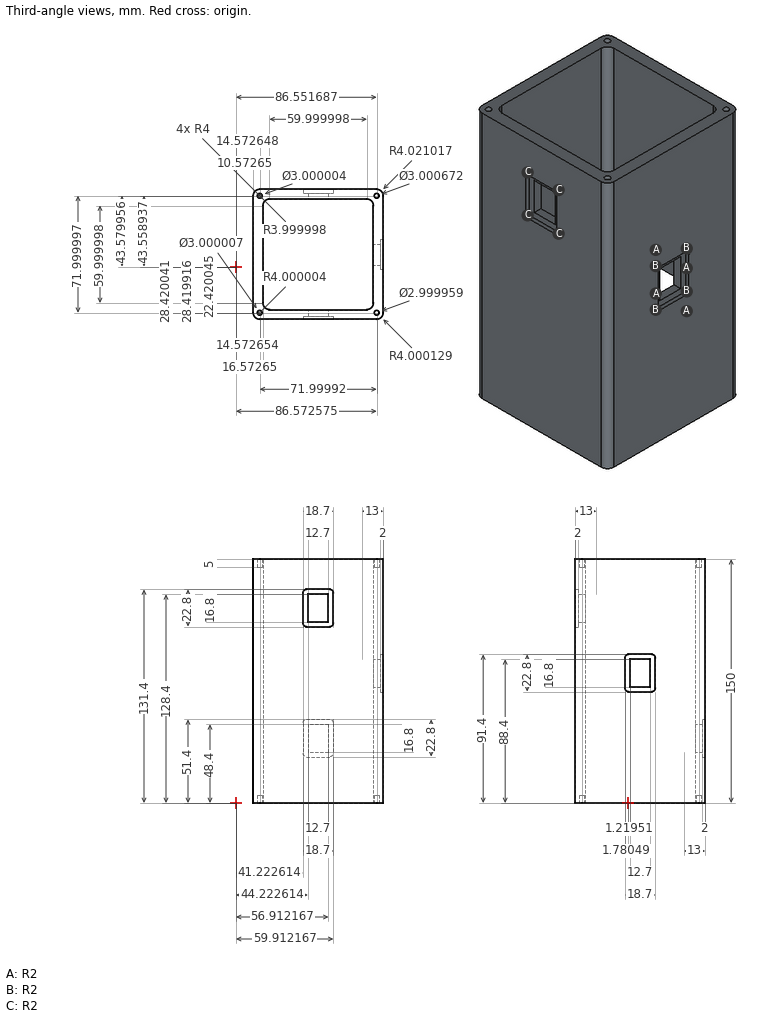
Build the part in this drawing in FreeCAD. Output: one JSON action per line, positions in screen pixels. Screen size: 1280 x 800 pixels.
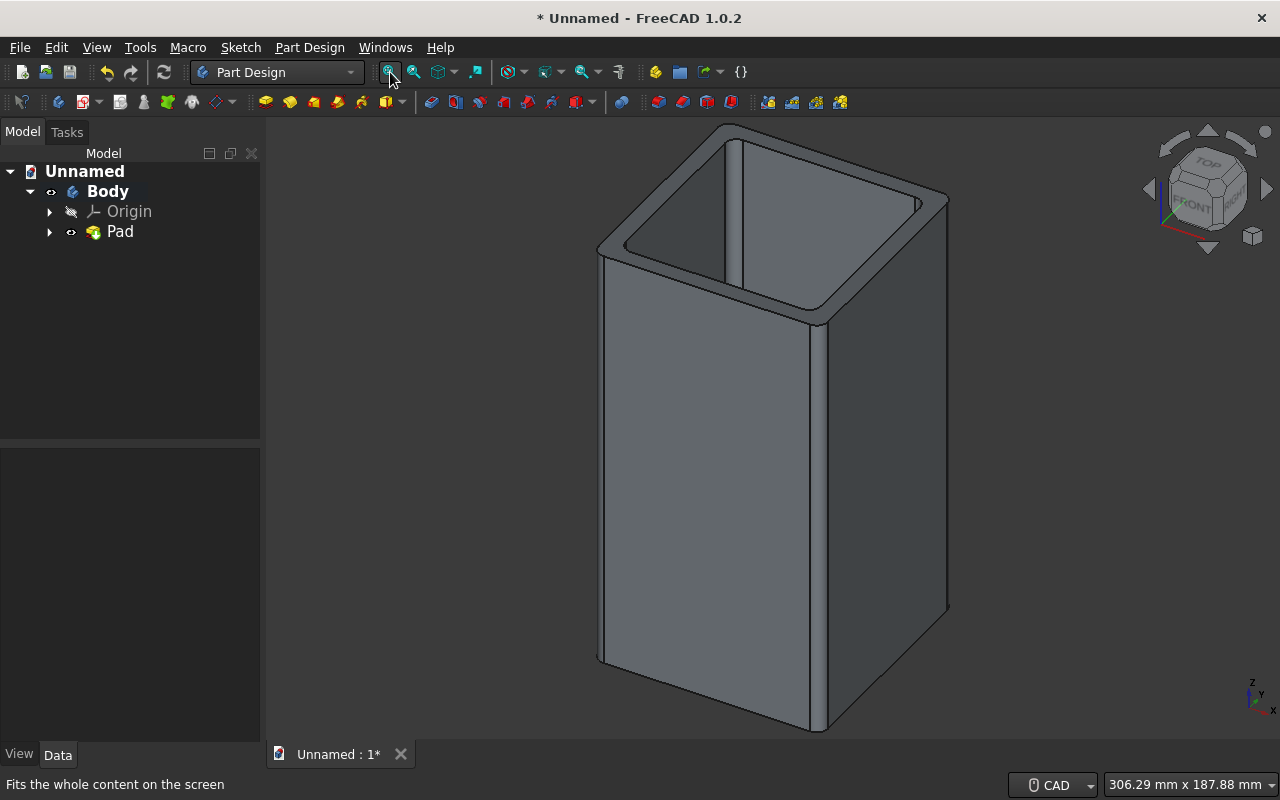
{"action": "left_click", "coordinate": [815, 313]}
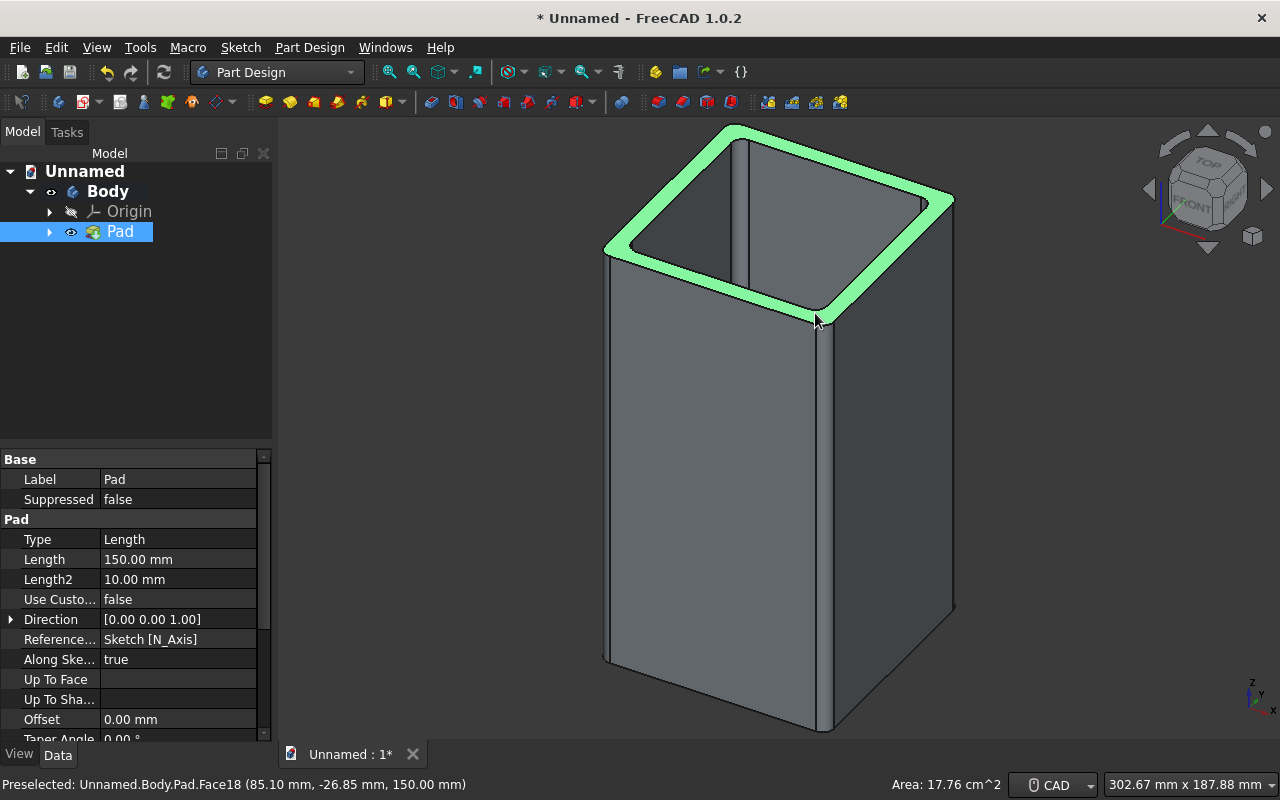
{"action": "left_click", "coordinate": [84, 102]}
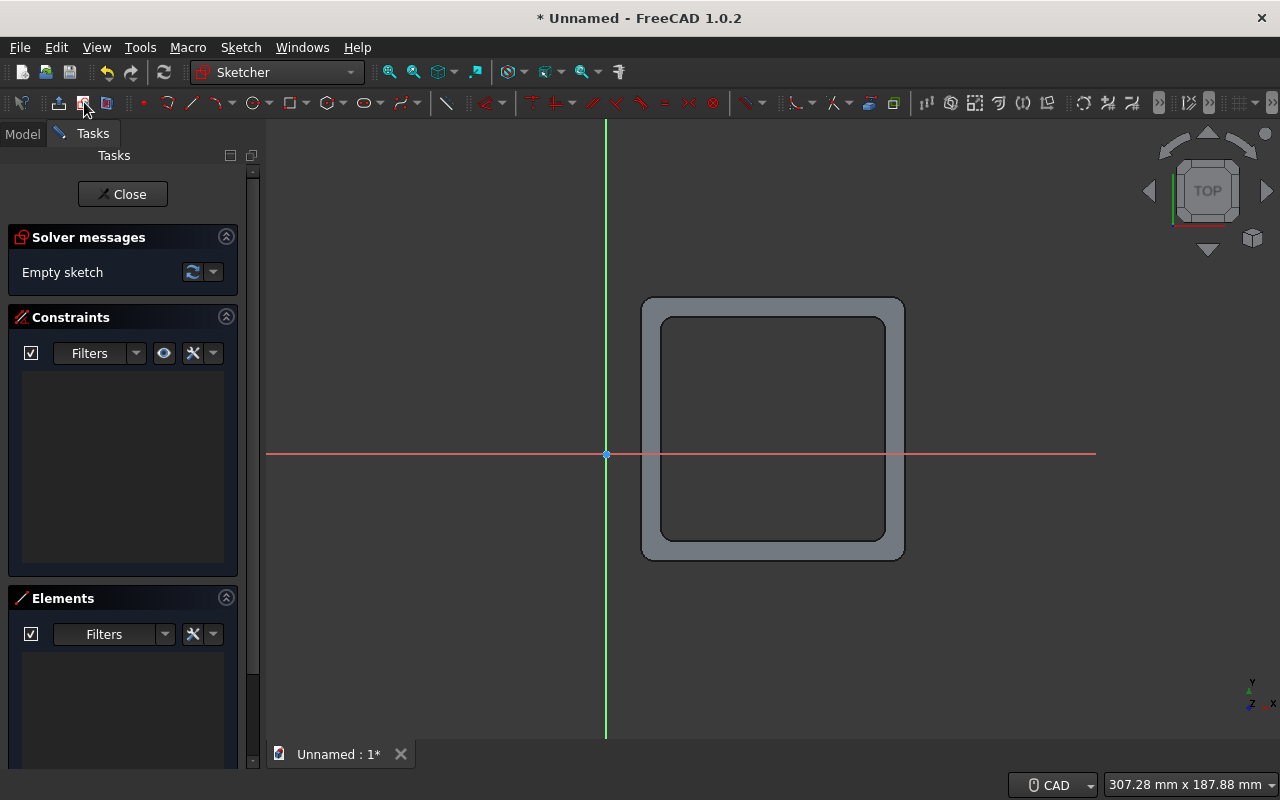
{"action": "scroll", "coordinate": [847, 429], "scroll_direction": "up", "scroll_amount": 2}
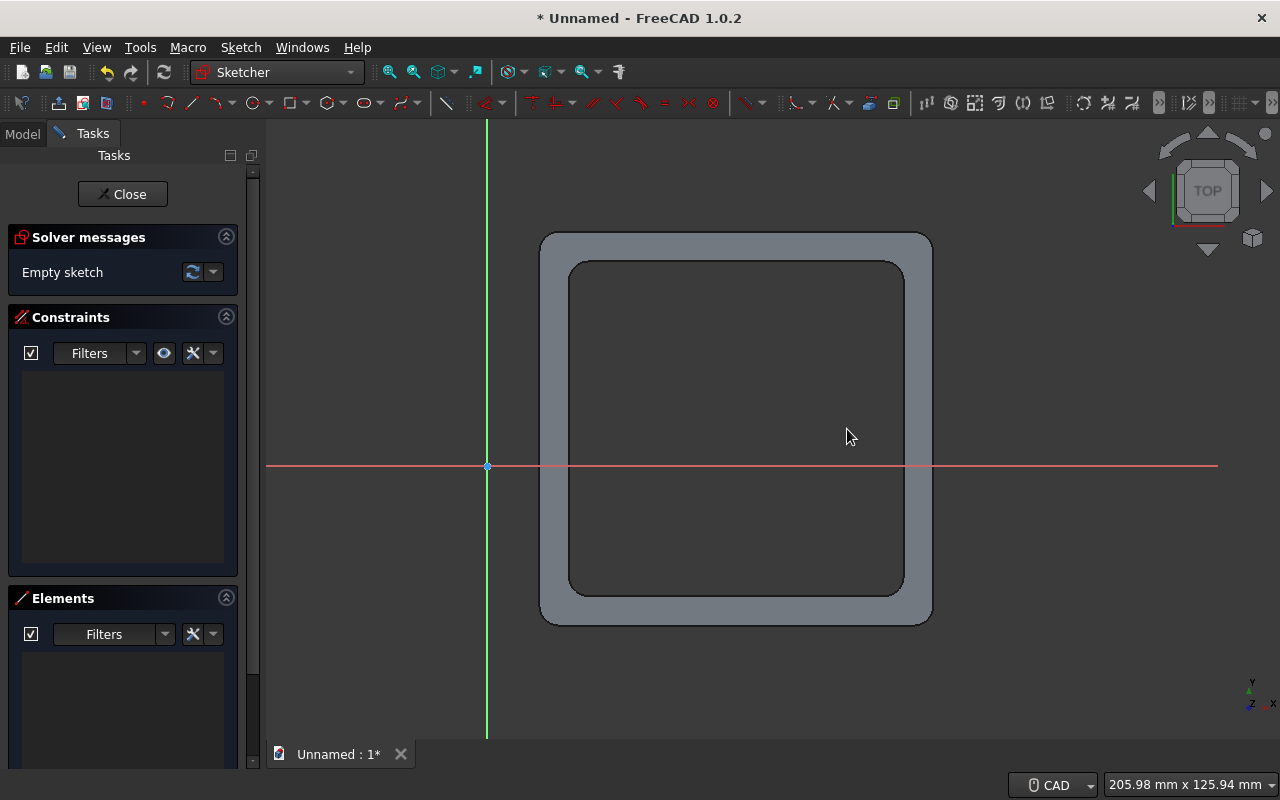
{"action": "left_click", "coordinate": [254, 104]}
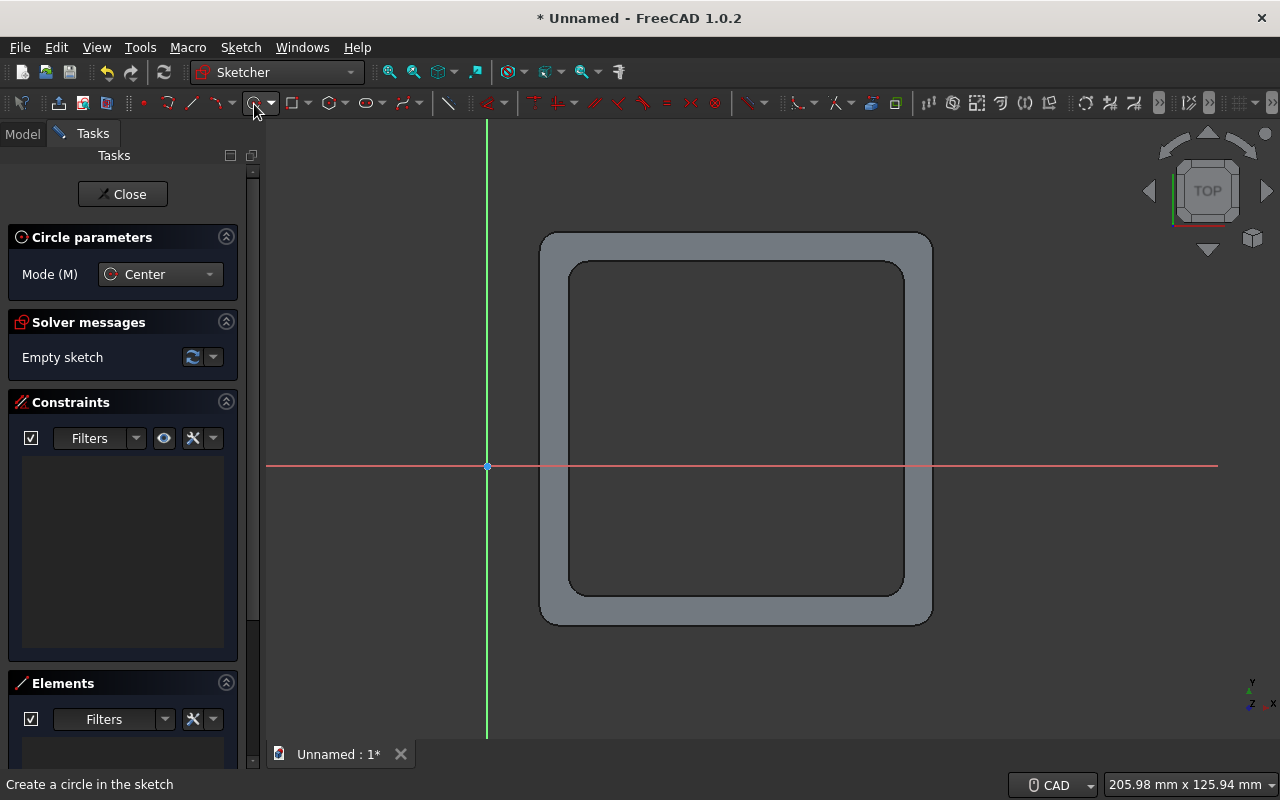
{"action": "scroll", "coordinate": [559, 606], "scroll_direction": "up", "scroll_amount": 6}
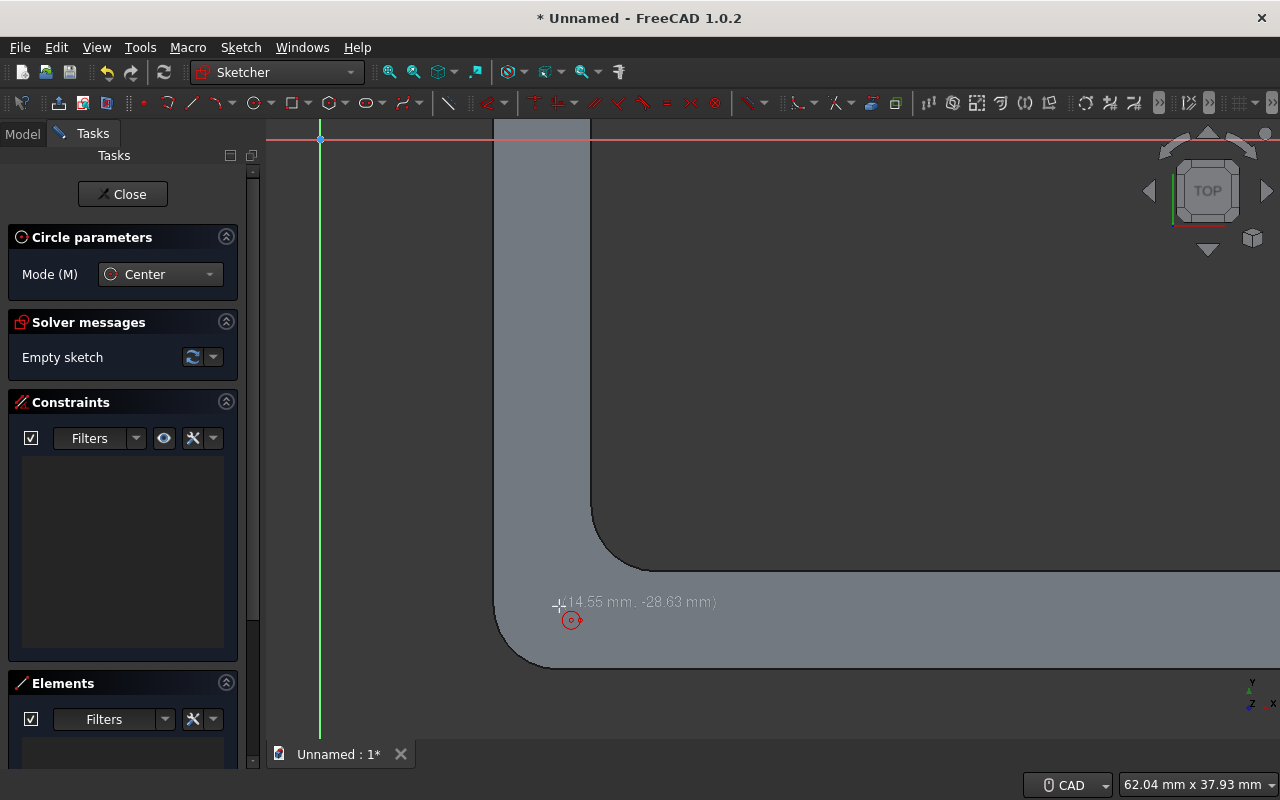
{"action": "left_click", "coordinate": [559, 604]}
{"action": "left_click", "coordinate": [576, 587]}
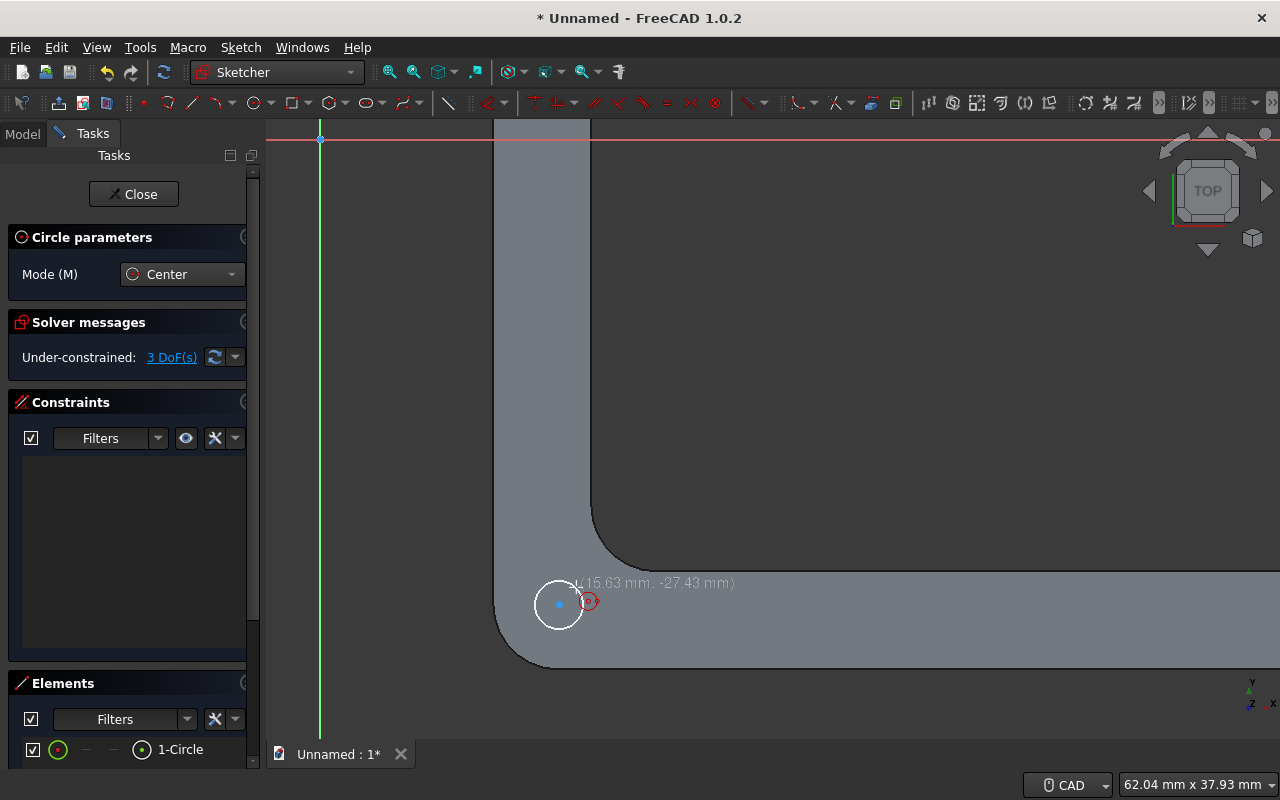
{"action": "scroll", "coordinate": [560, 607], "scroll_direction": "down", "scroll_amount": 6}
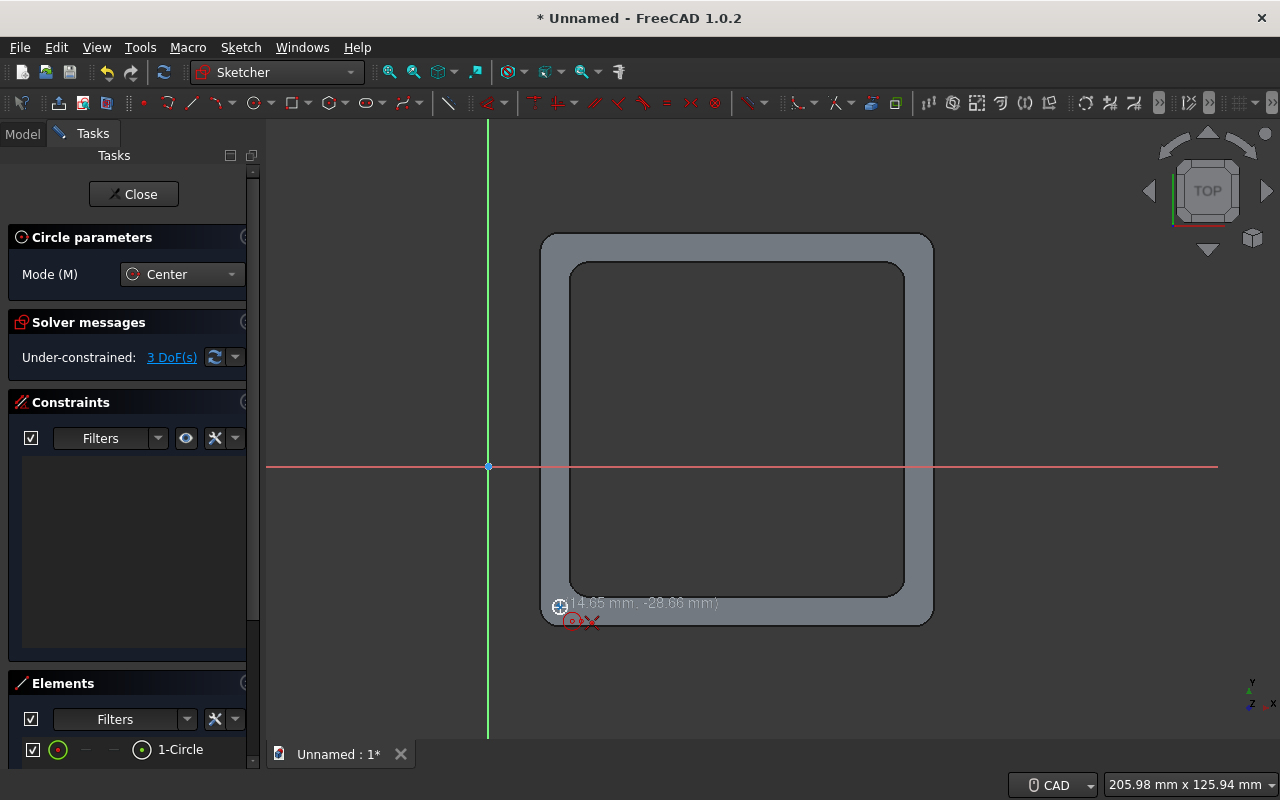
{"action": "scroll", "coordinate": [560, 252], "scroll_direction": "up", "scroll_amount": 6}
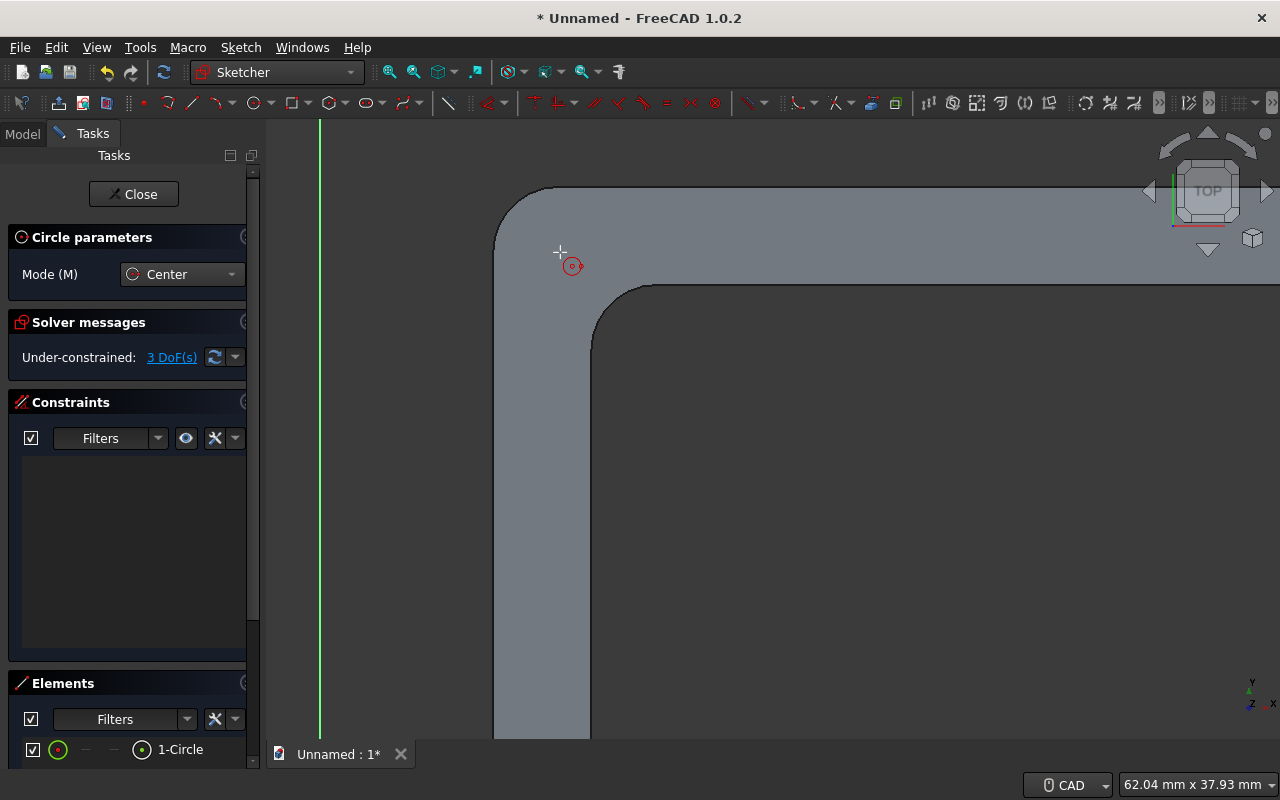
{"action": "left_click", "coordinate": [559, 252]}
{"action": "left_click", "coordinate": [576, 235]}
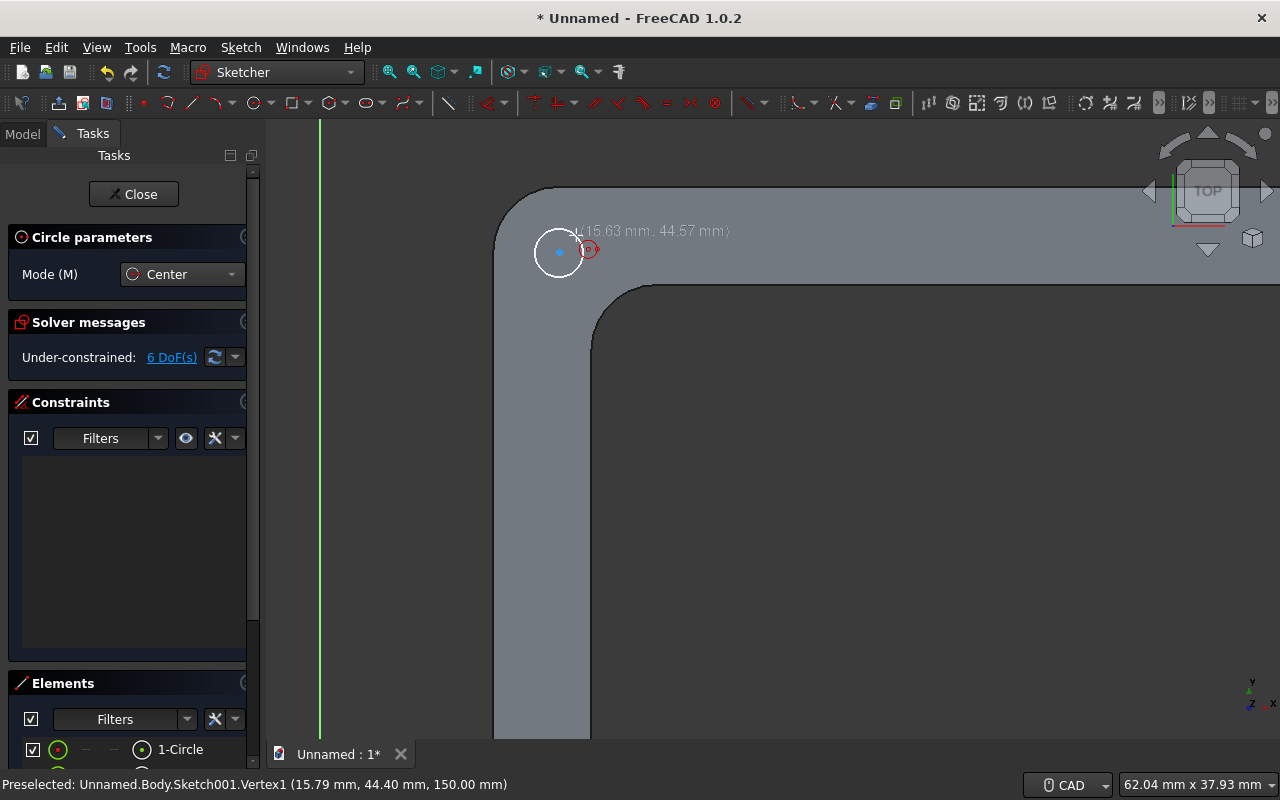
{"action": "scroll", "coordinate": [560, 252], "scroll_direction": "down", "scroll_amount": 6}